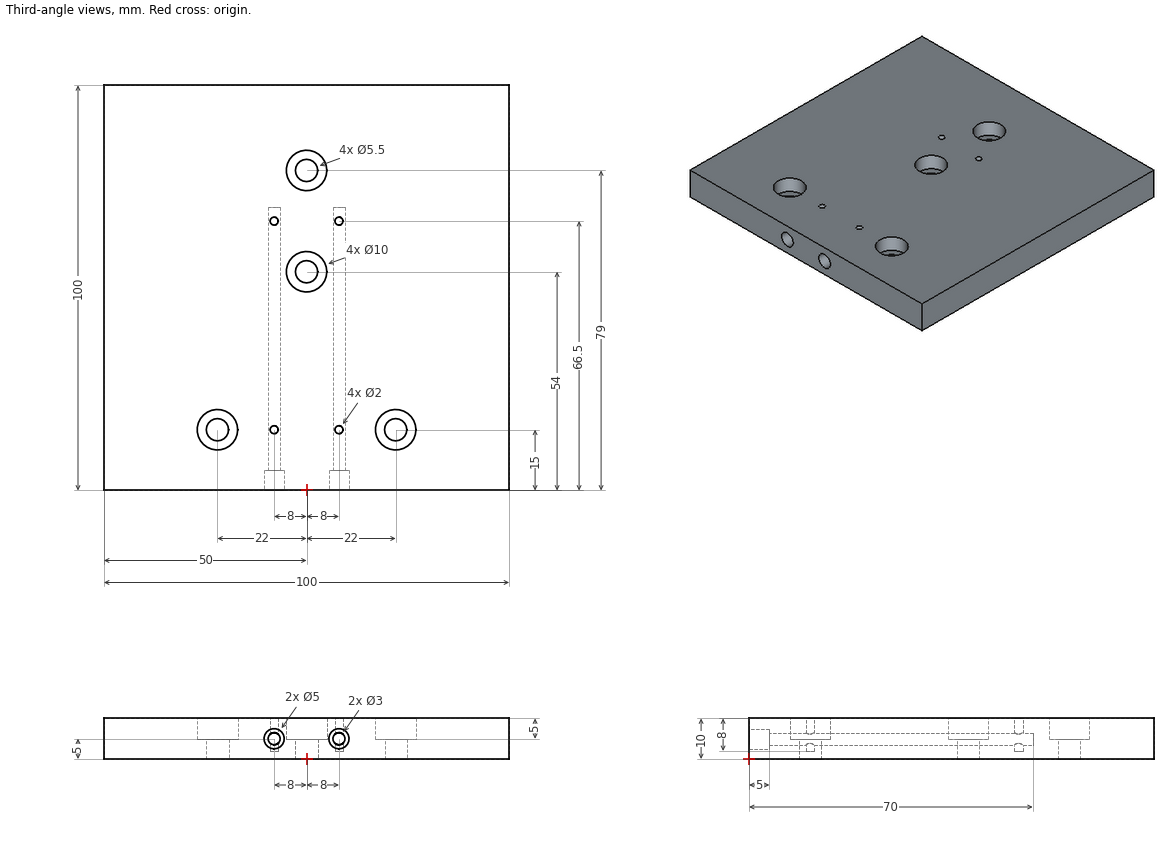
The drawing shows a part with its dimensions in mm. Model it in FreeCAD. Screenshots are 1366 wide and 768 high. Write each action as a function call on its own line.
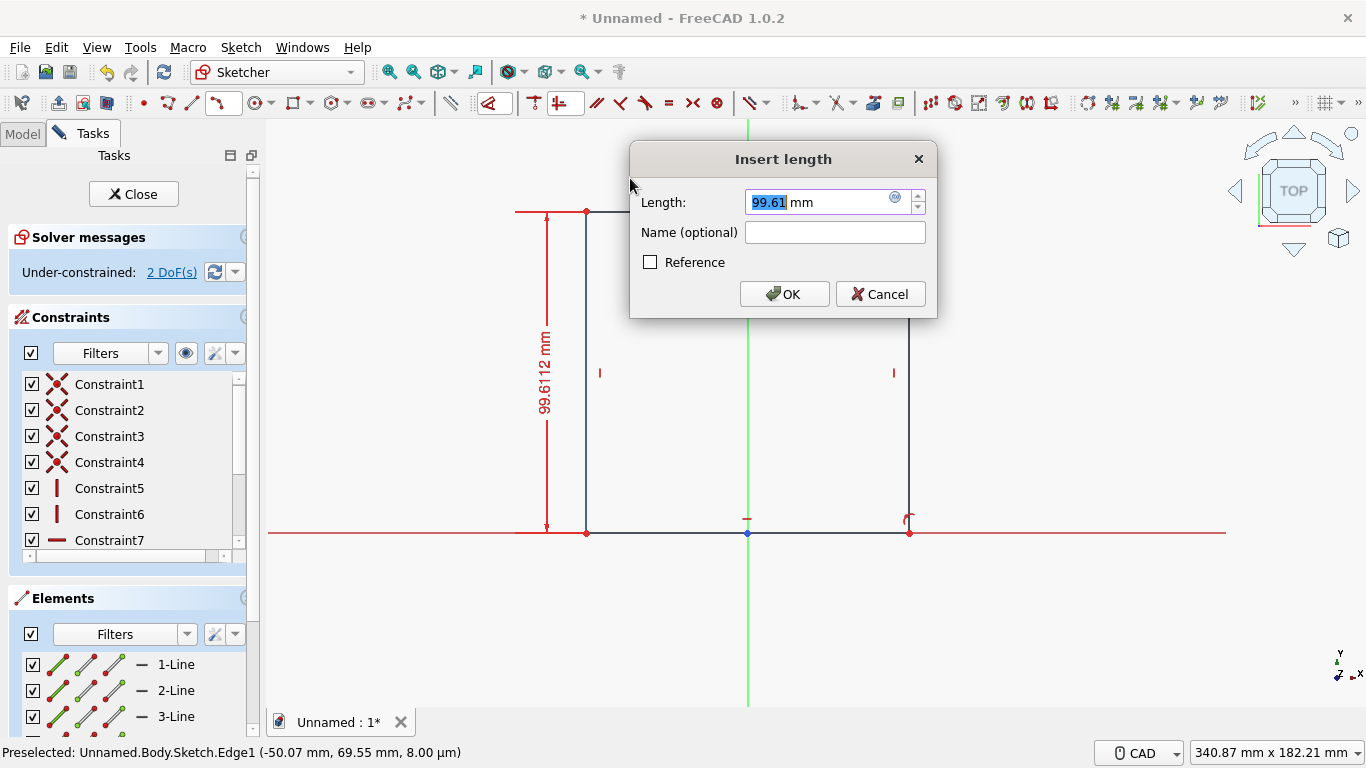
text(100)
key(Return)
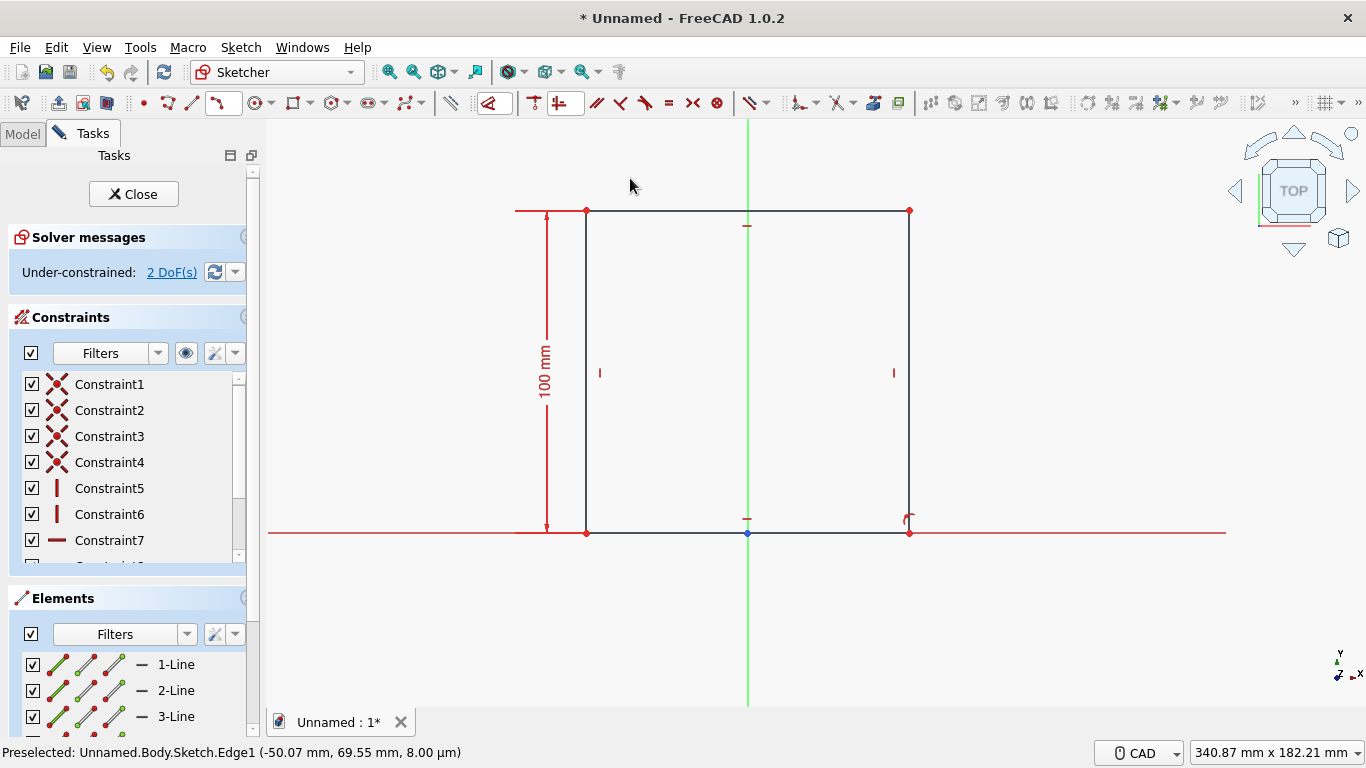
click(683, 533)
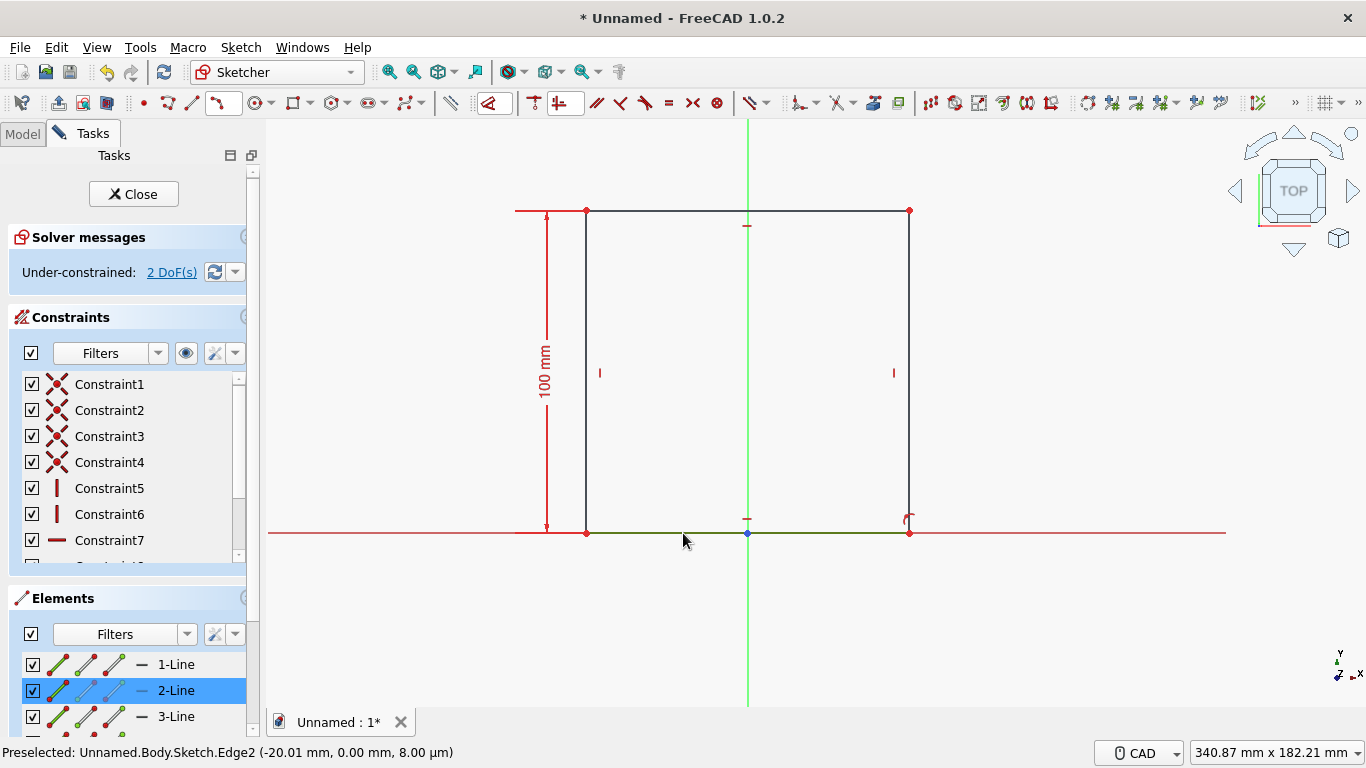
click(506, 104)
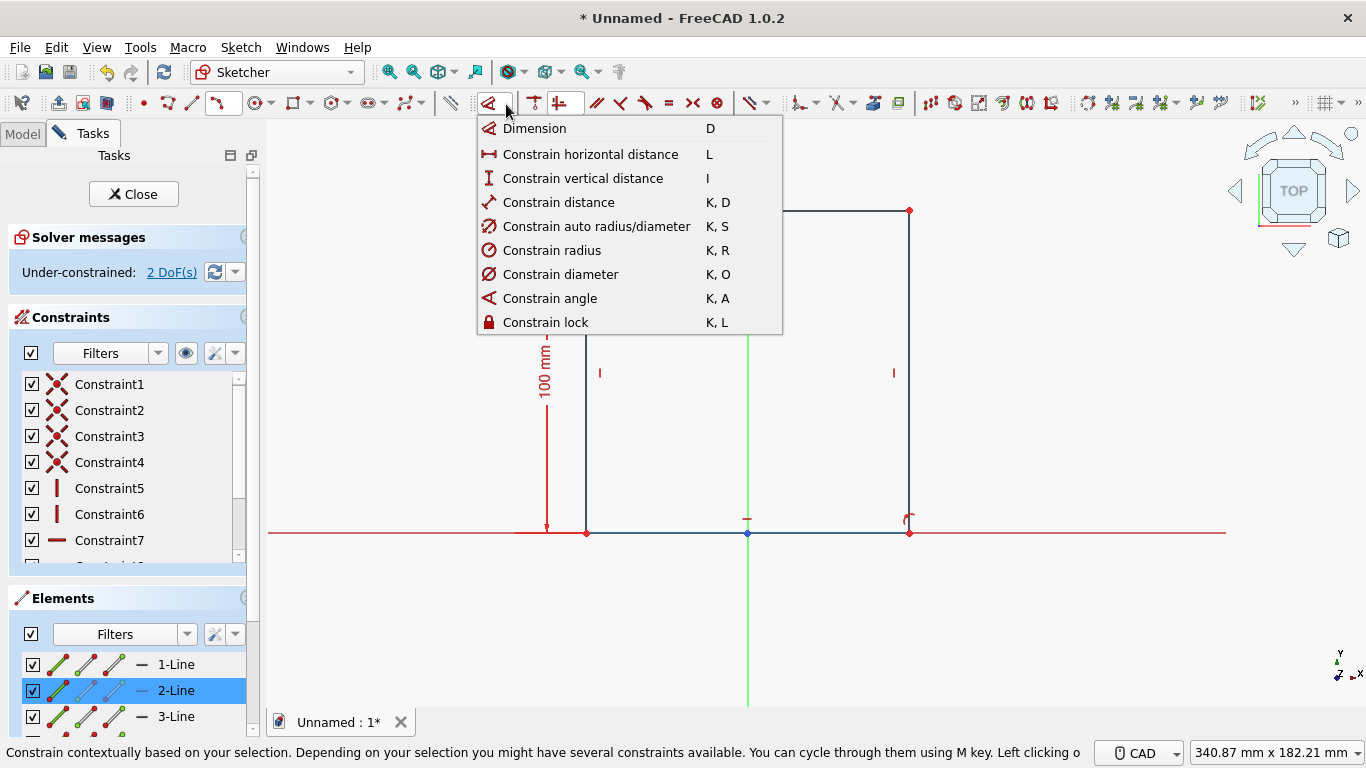
click(630, 154)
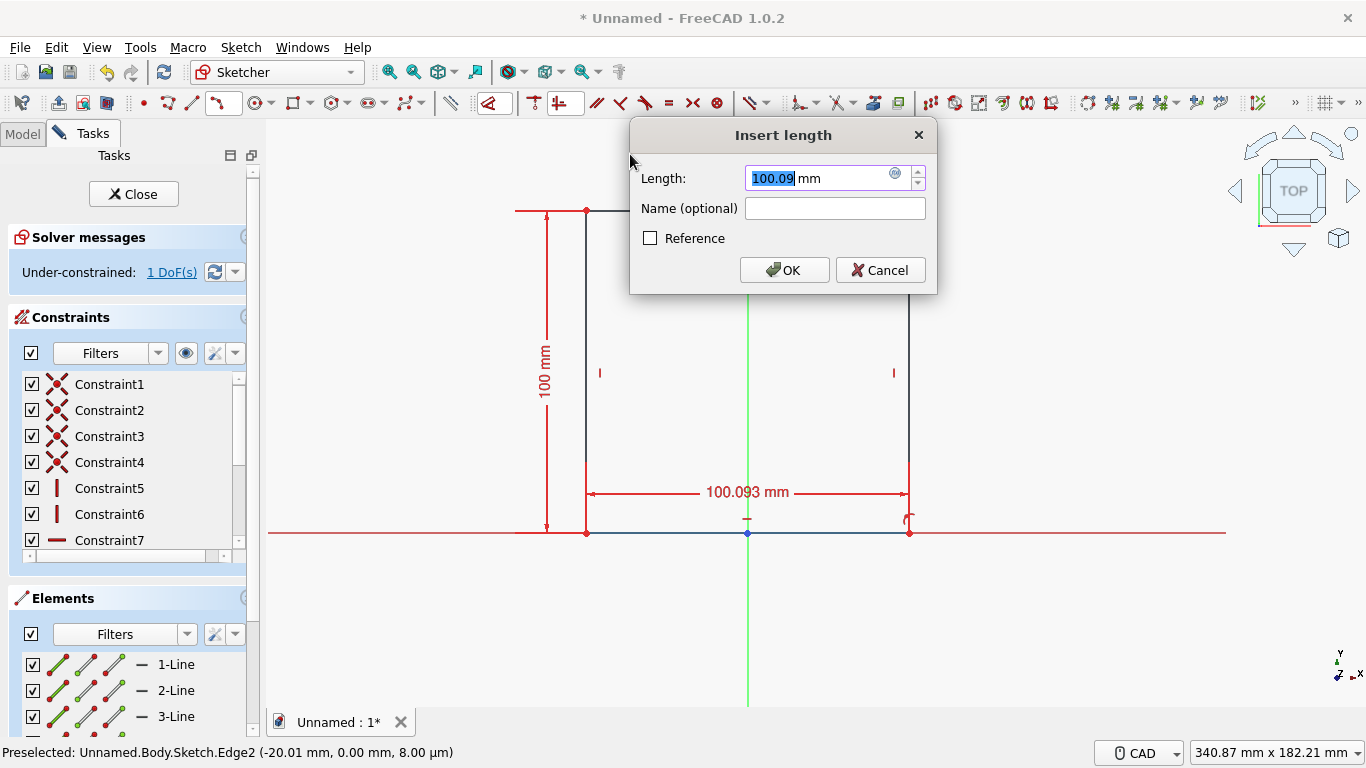
text(100)
key(Return)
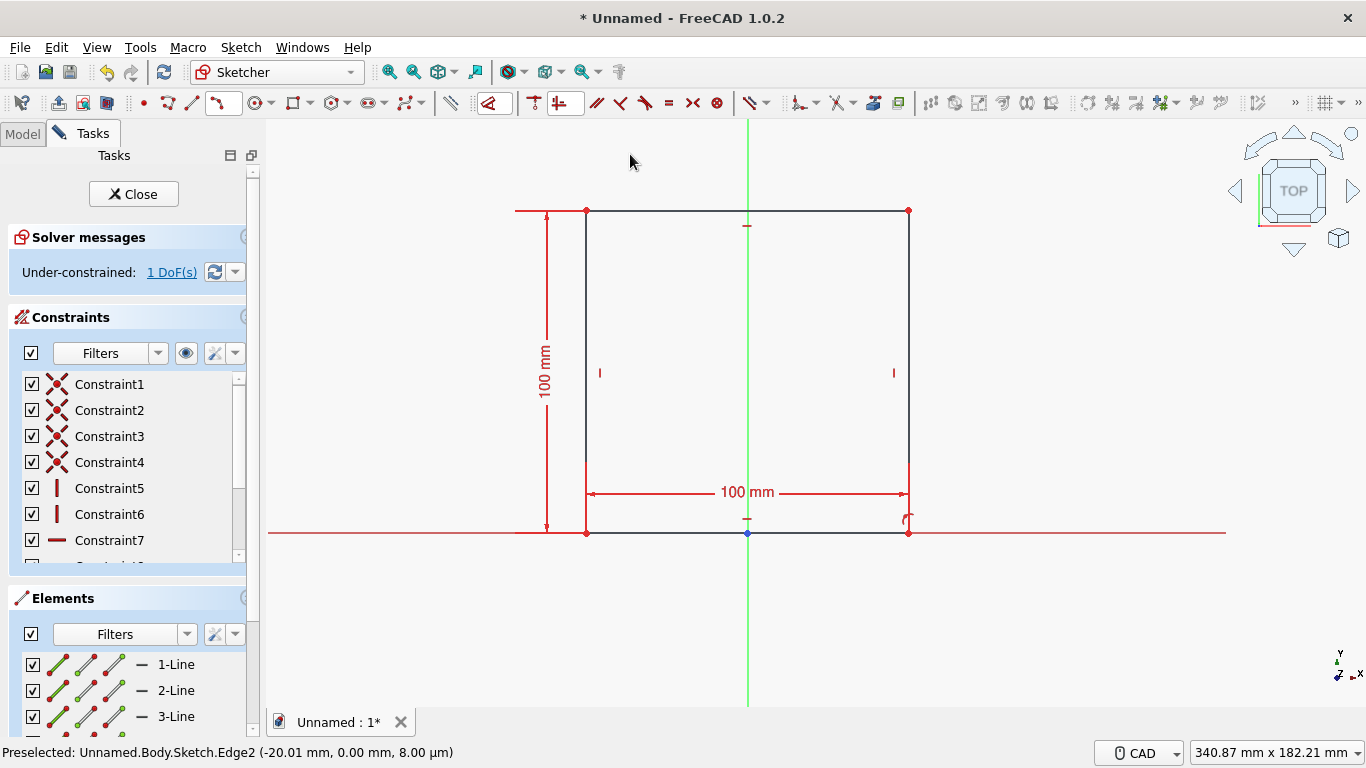
click(586, 211)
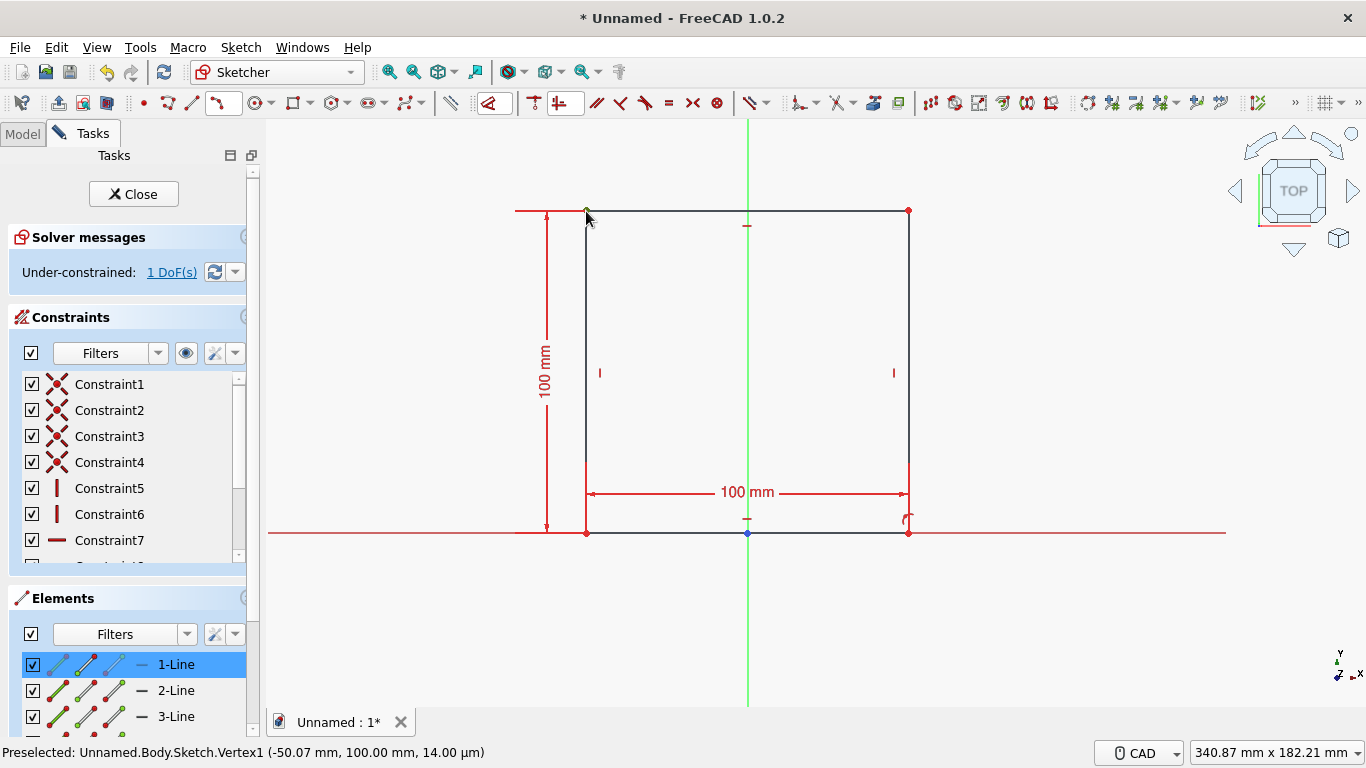
click(506, 104)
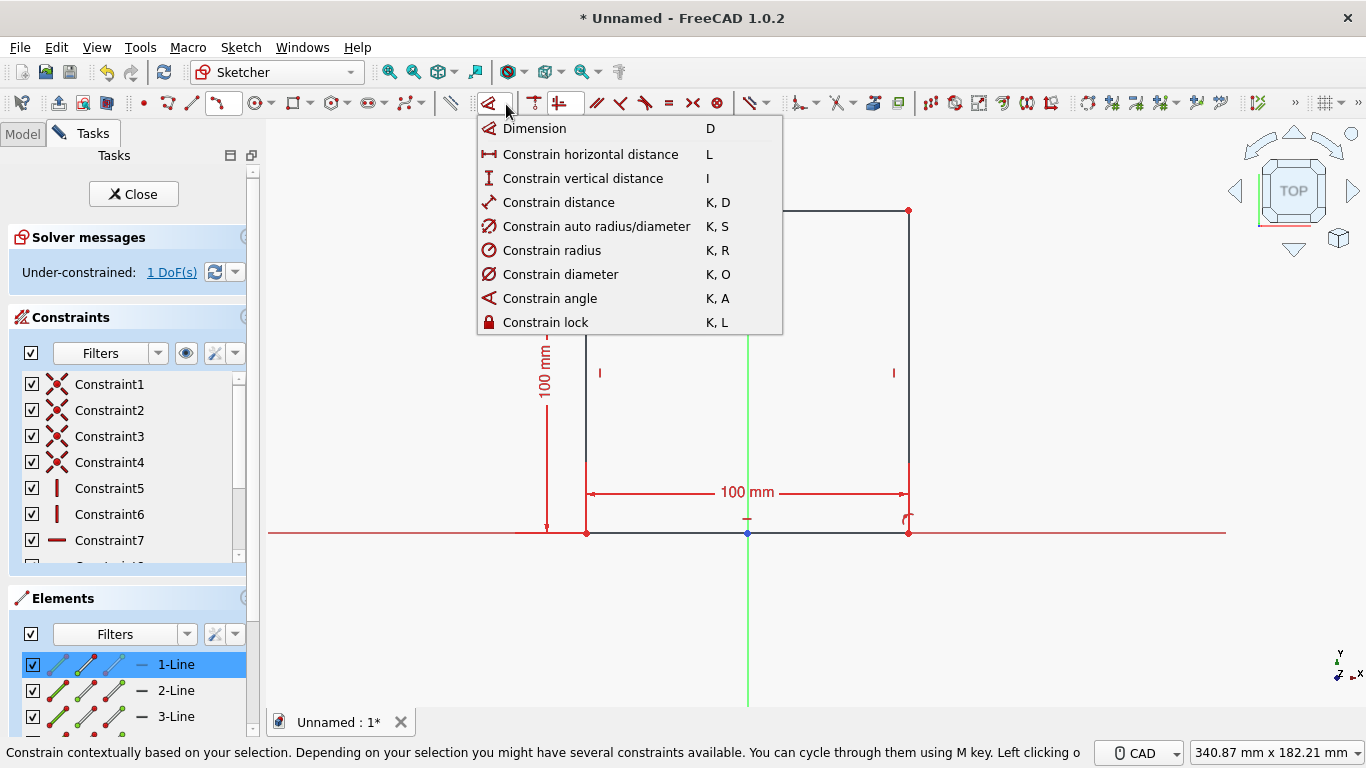
click(630, 154)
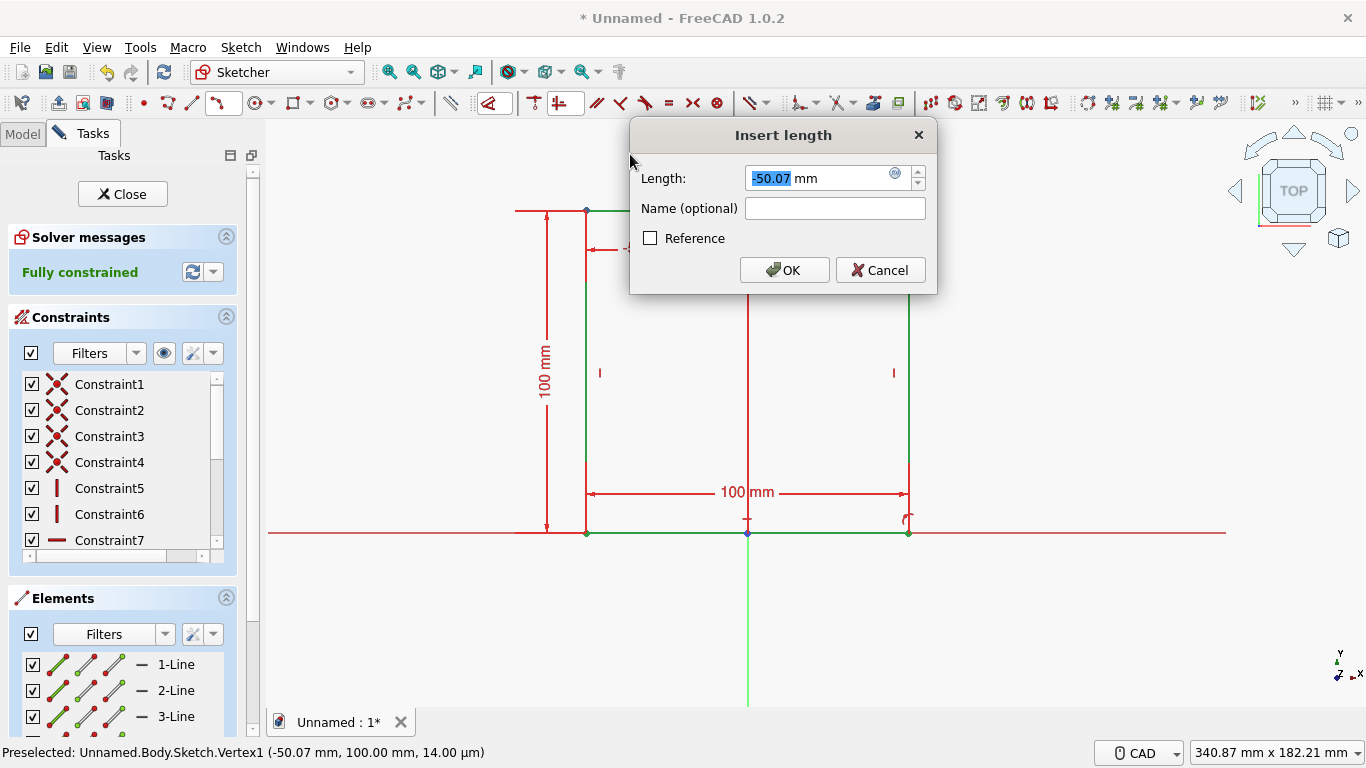
text(-50)
key(Return)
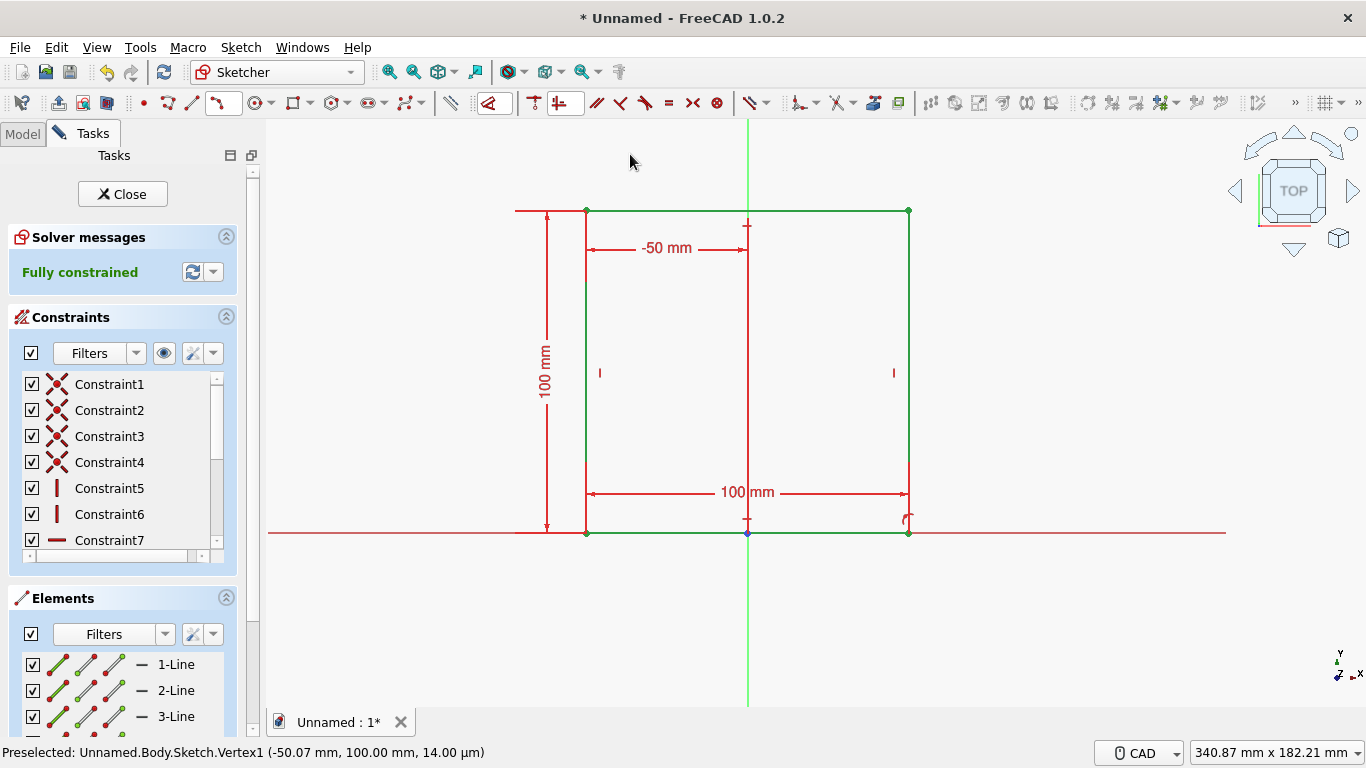
click(123, 194)